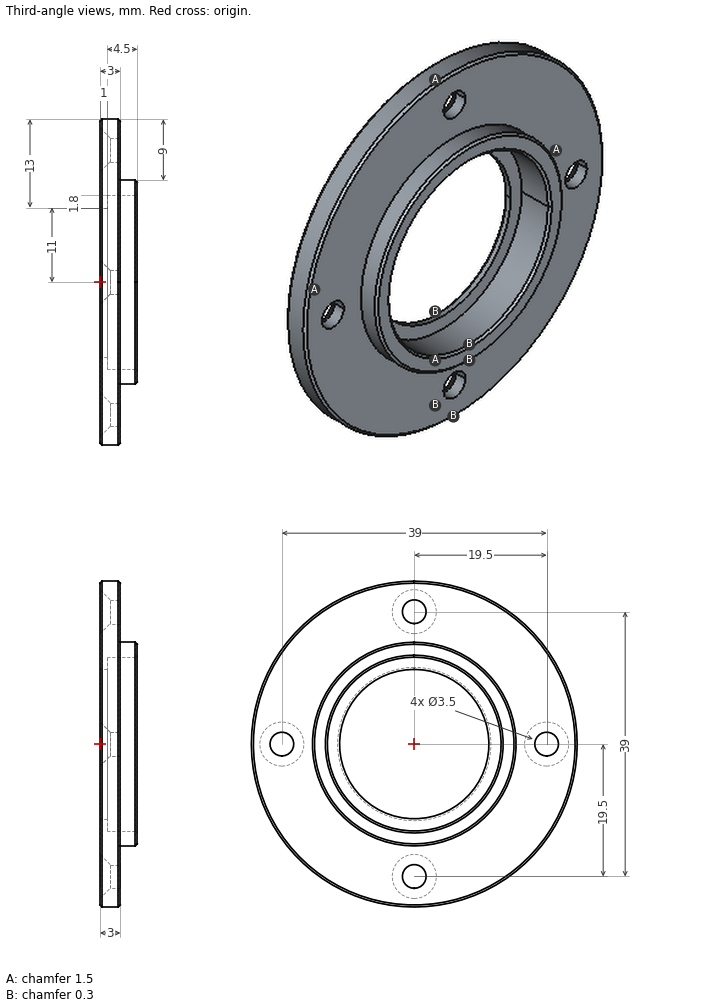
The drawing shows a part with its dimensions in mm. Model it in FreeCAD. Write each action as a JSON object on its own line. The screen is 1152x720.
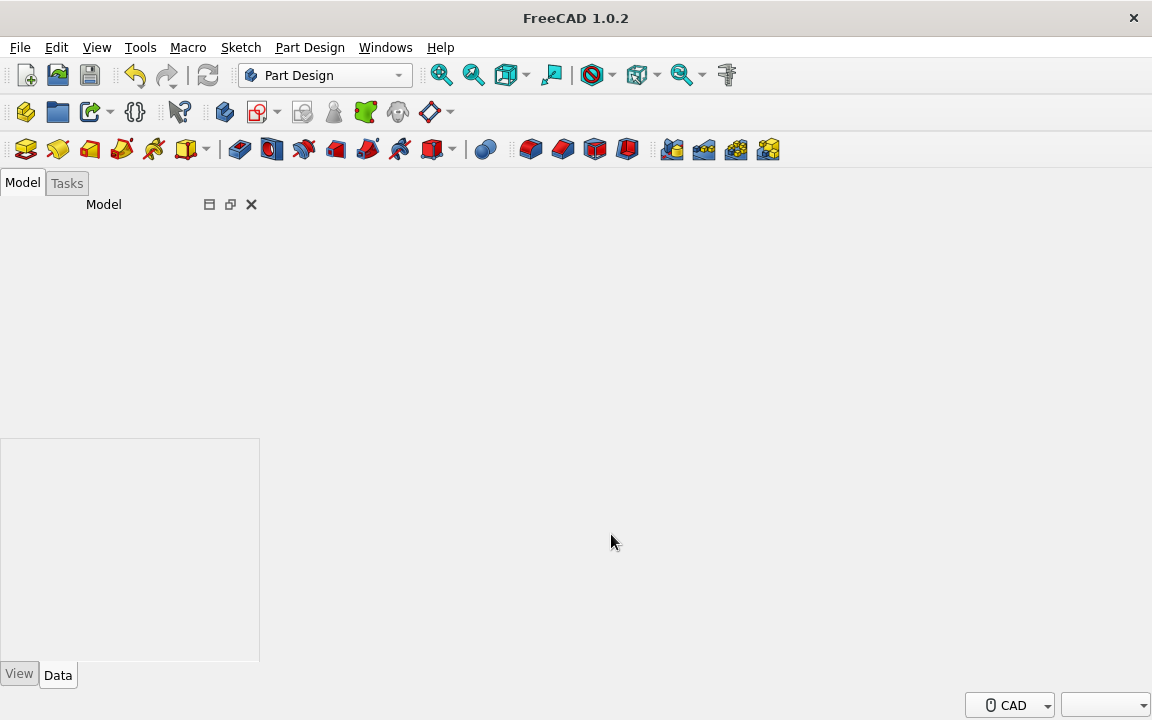
{"action": "left_click", "coordinate": [26, 76]}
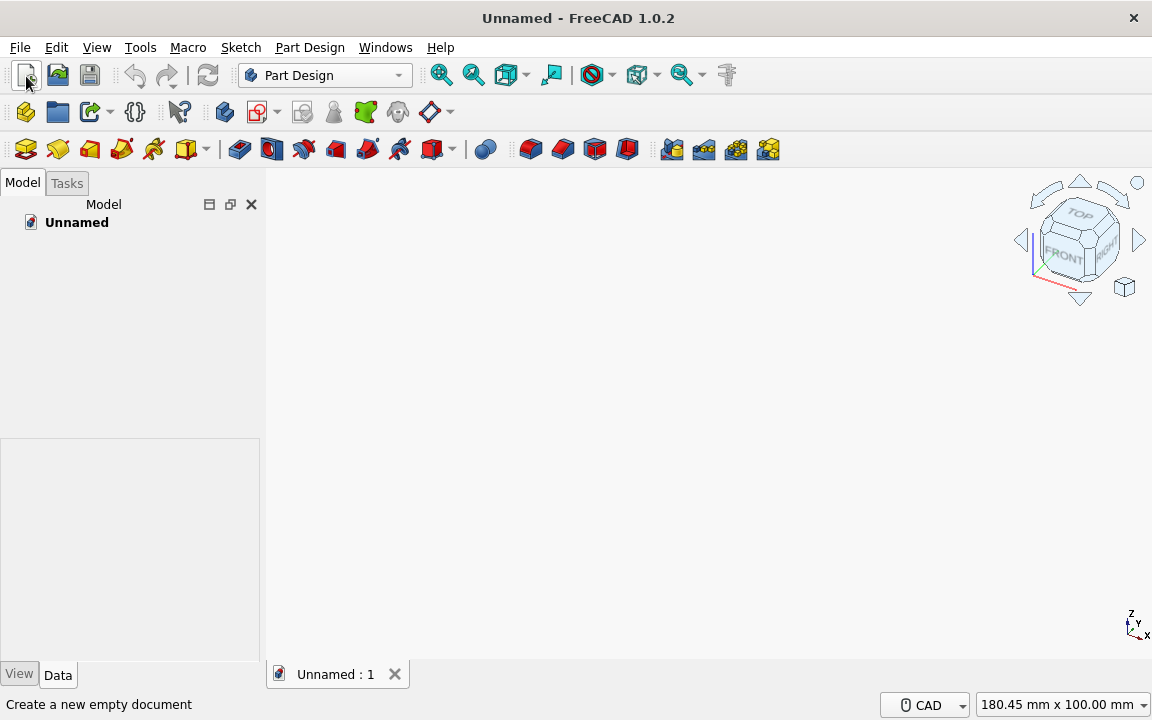
{"action": "left_click", "coordinate": [258, 112]}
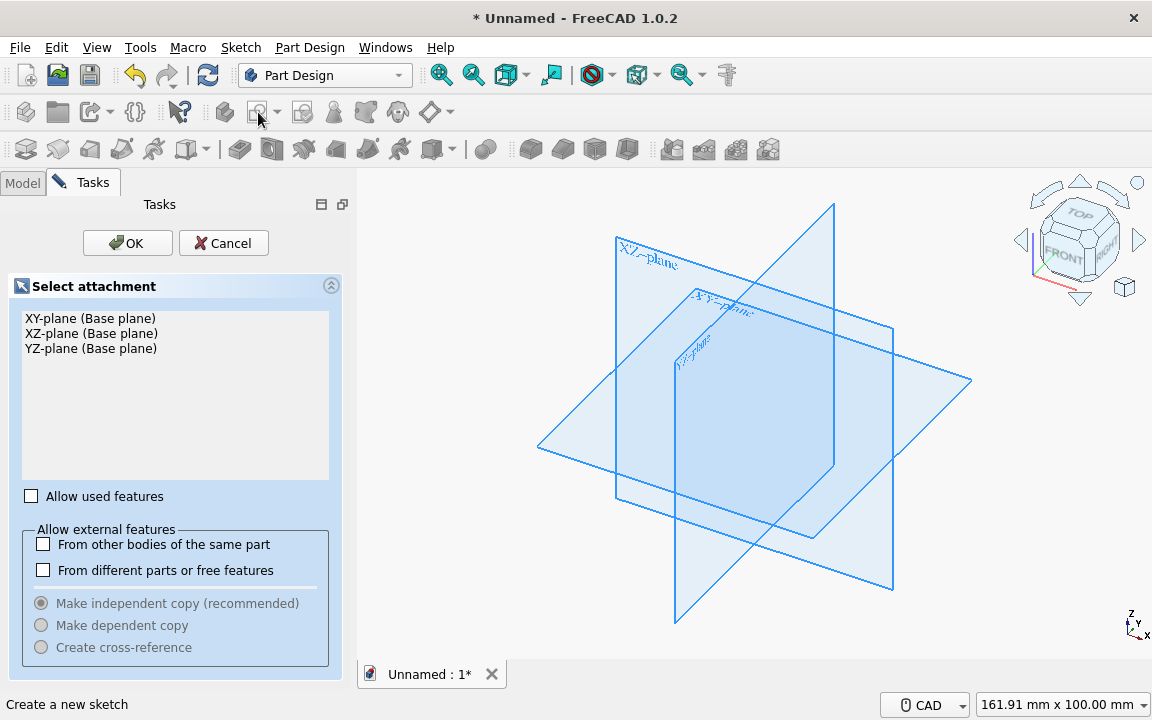
{"action": "left_click", "coordinate": [82, 318]}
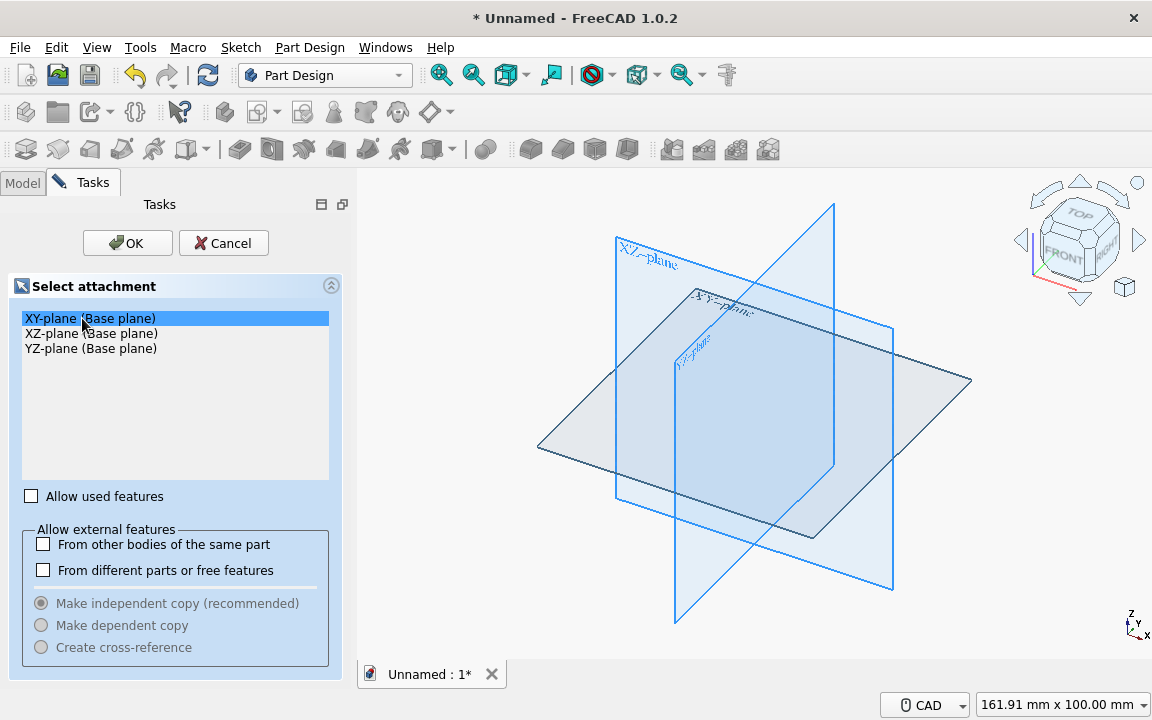
{"action": "left_click", "coordinate": [128, 243]}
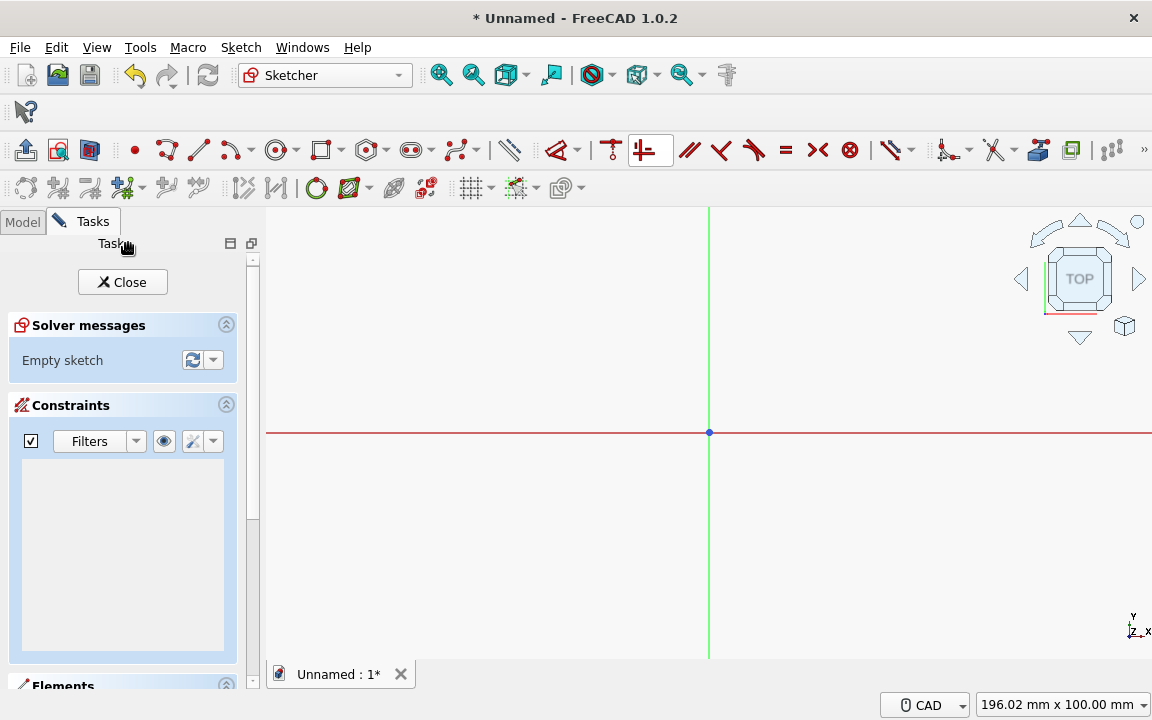
{"action": "scroll", "coordinate": [769, 347], "scroll_direction": "up", "scroll_amount": 5}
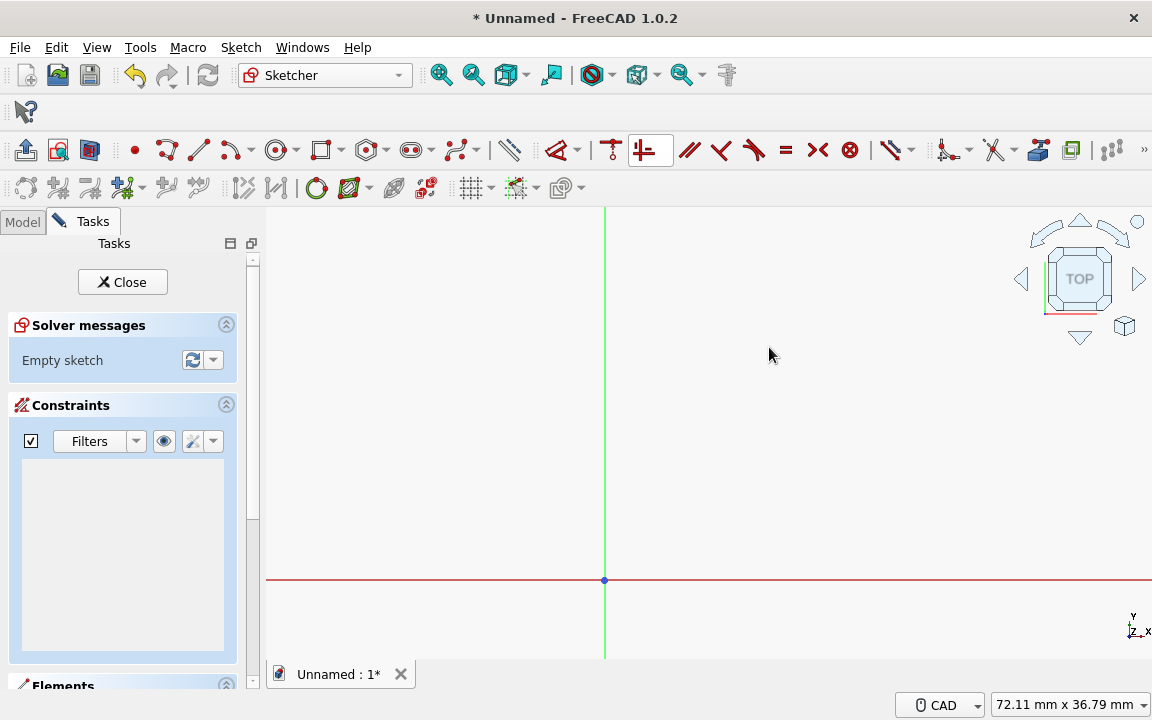
{"action": "left_click", "coordinate": [168, 150]}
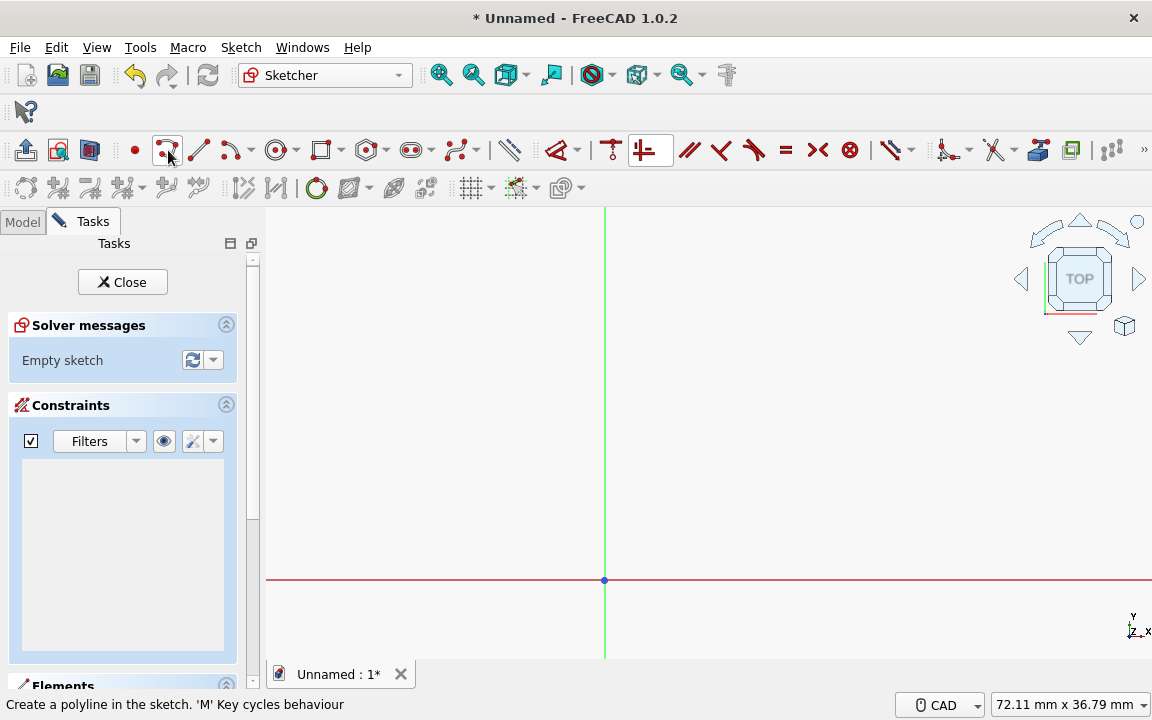
{"action": "left_click", "coordinate": [605, 445]}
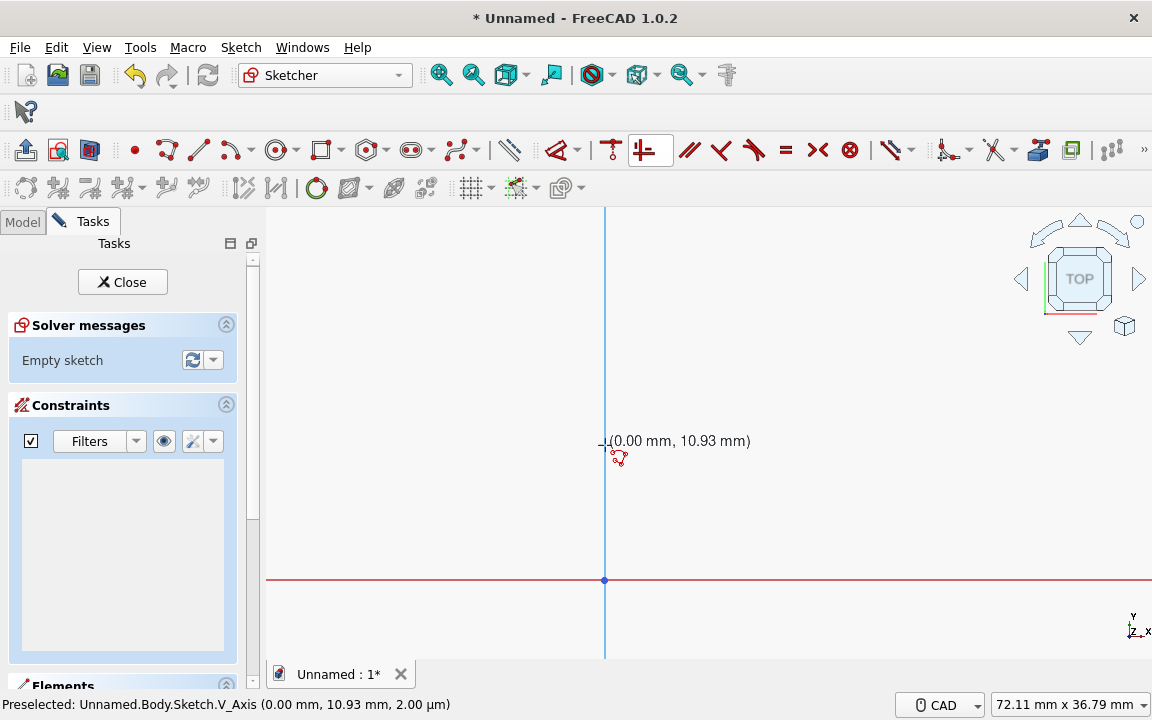
{"action": "scroll", "coordinate": [617, 445], "scroll_direction": "up", "scroll_amount": 2}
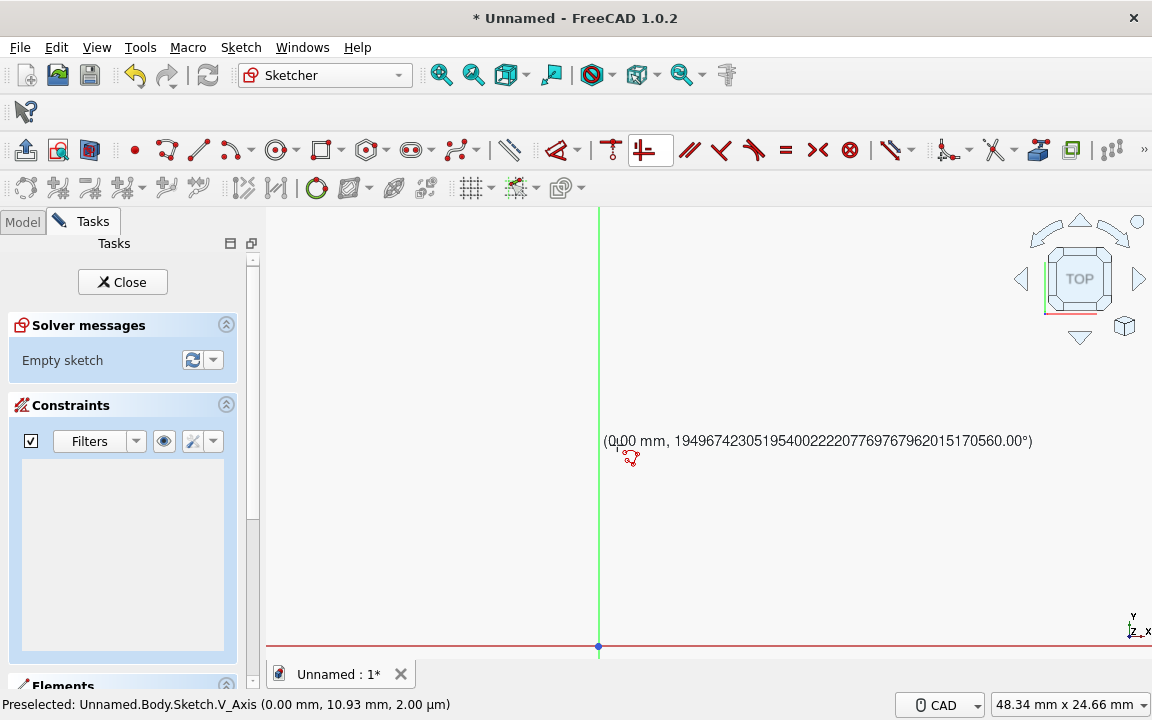
{"action": "left_click", "coordinate": [617, 445]}
{"action": "left_click", "coordinate": [617, 412]}
{"action": "left_click", "coordinate": [700, 412]}
{"action": "left_click", "coordinate": [700, 372]}
{"action": "left_click", "coordinate": [654, 372]}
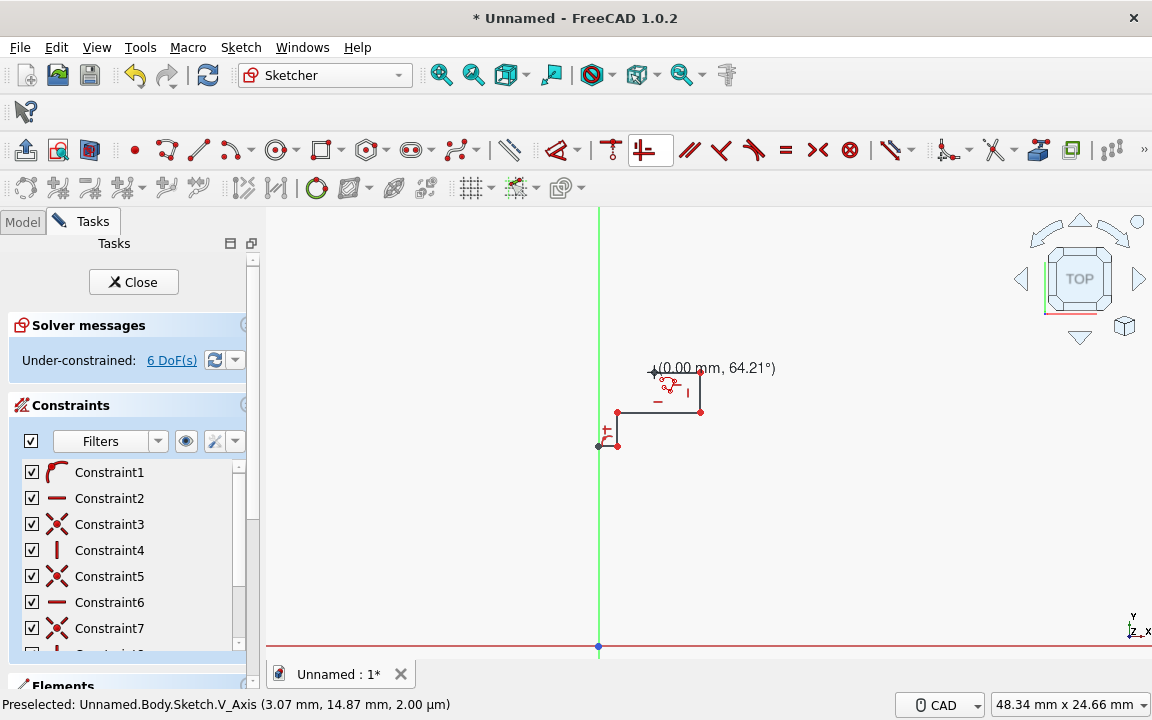
{"action": "scroll", "coordinate": [623, 446], "scroll_direction": "down", "scroll_amount": 2}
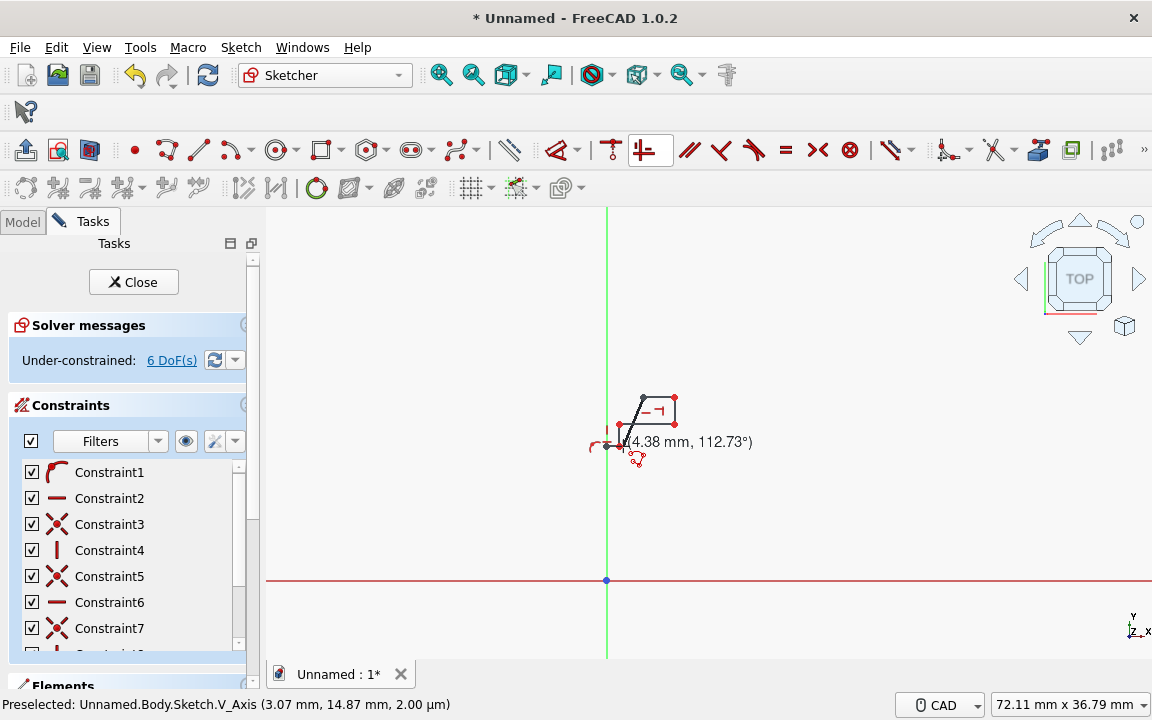
{"action": "left_click", "coordinate": [644, 286]}
{"action": "left_click", "coordinate": [616, 286]}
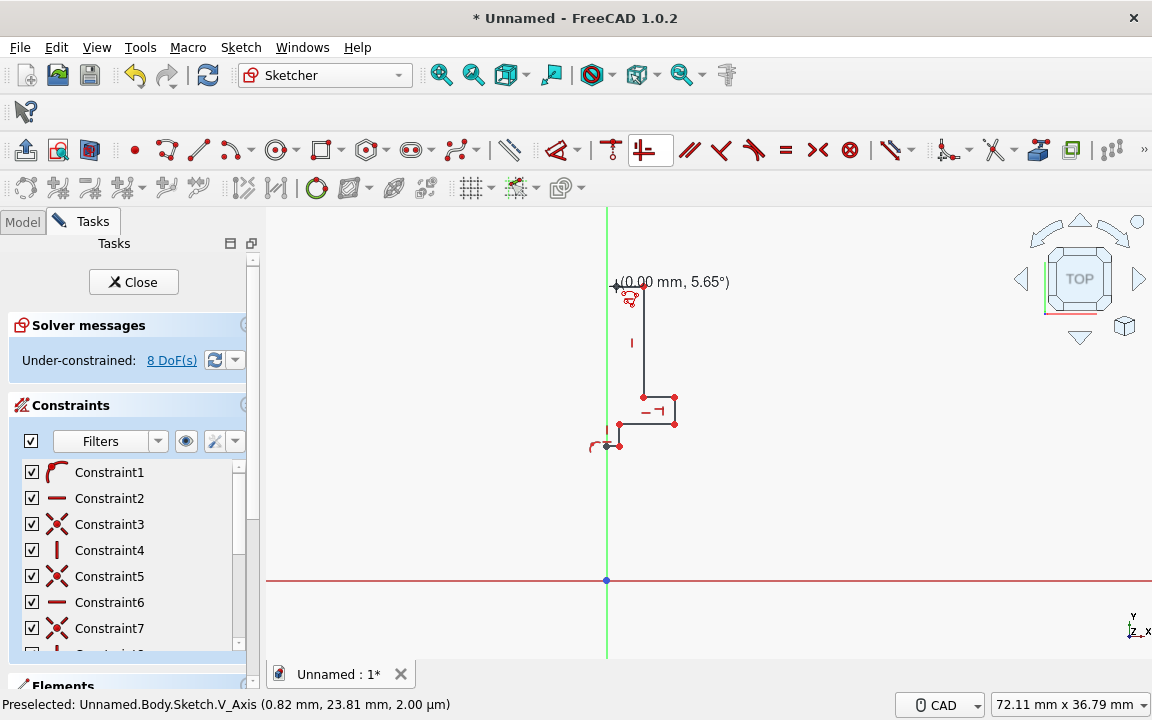
{"action": "scroll", "coordinate": [607, 445], "scroll_direction": "up", "scroll_amount": 5}